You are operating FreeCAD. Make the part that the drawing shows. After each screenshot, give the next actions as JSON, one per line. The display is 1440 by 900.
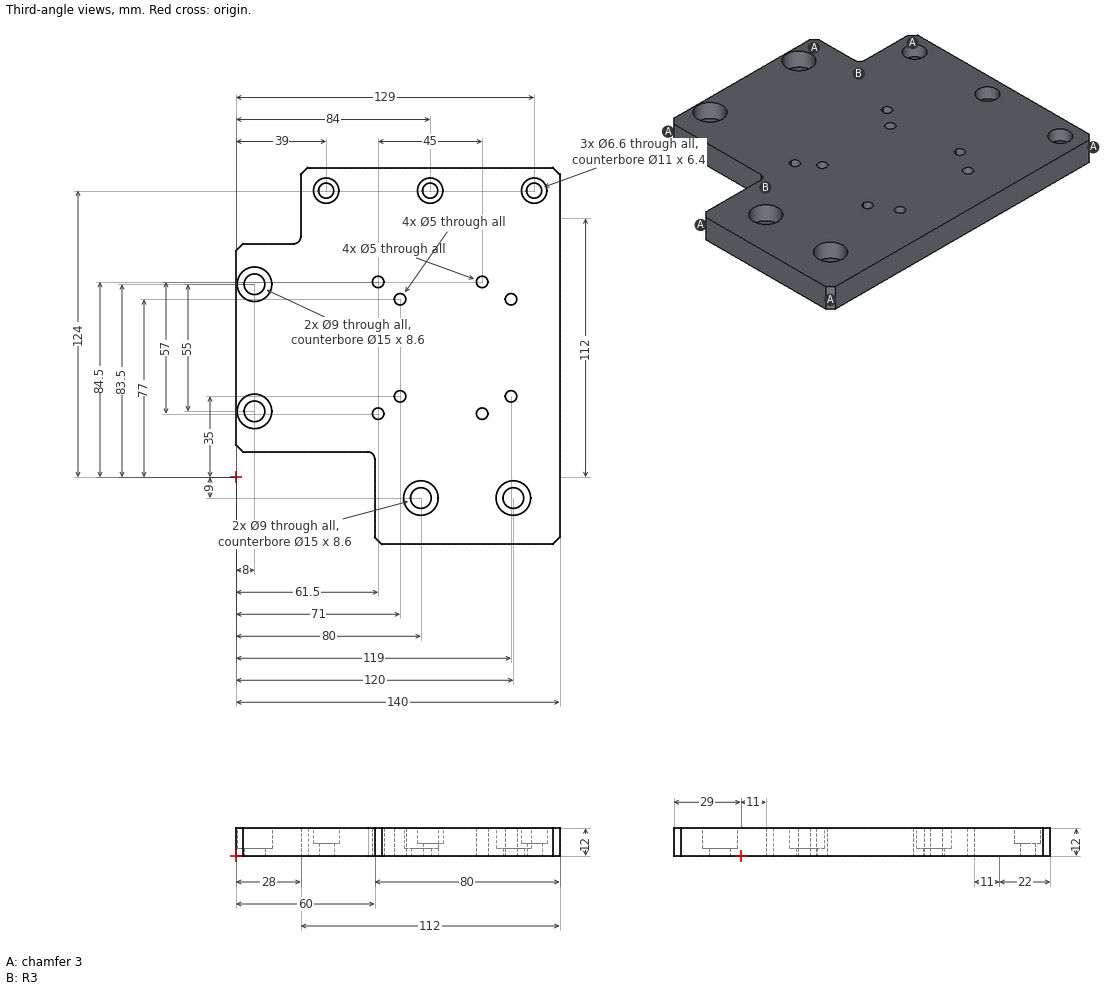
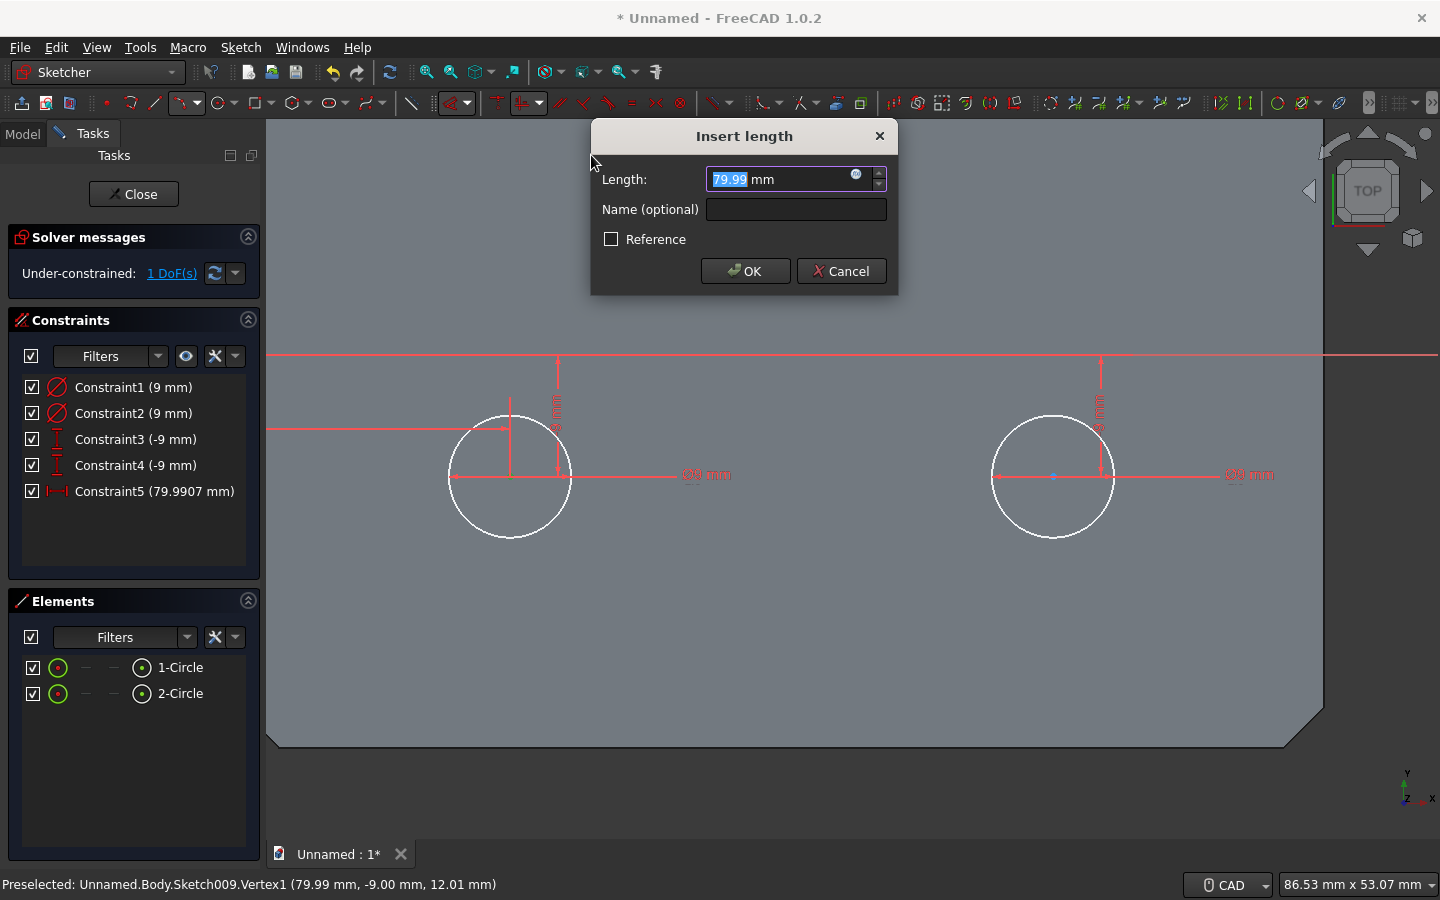
{"action": "type", "text": "80"}
{"action": "key", "text": "Return"}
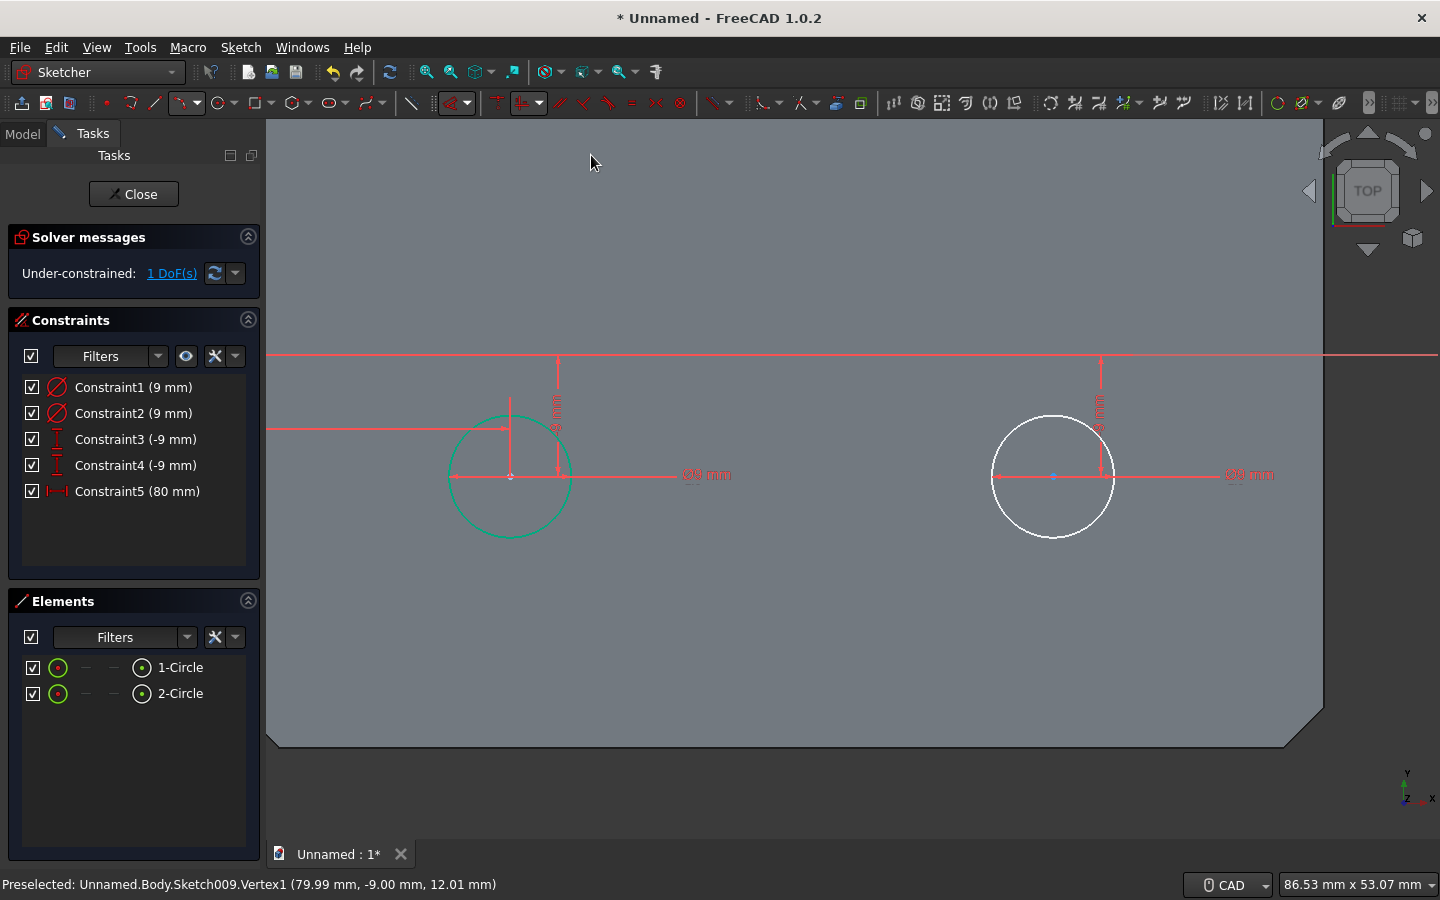
{"action": "left_click", "coordinate": [1053, 477]}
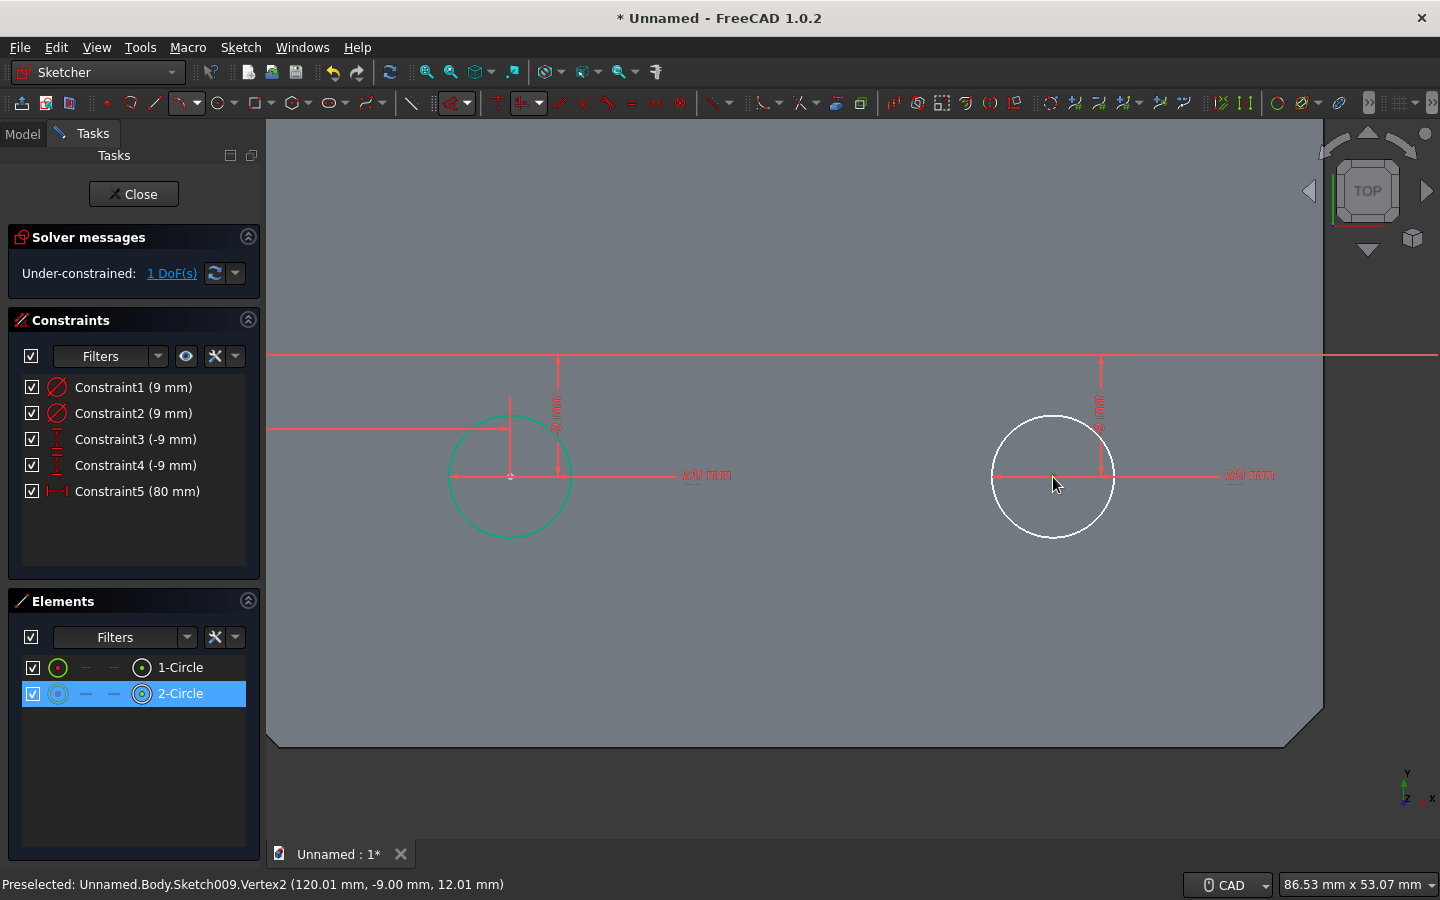
{"action": "key", "text": "l"}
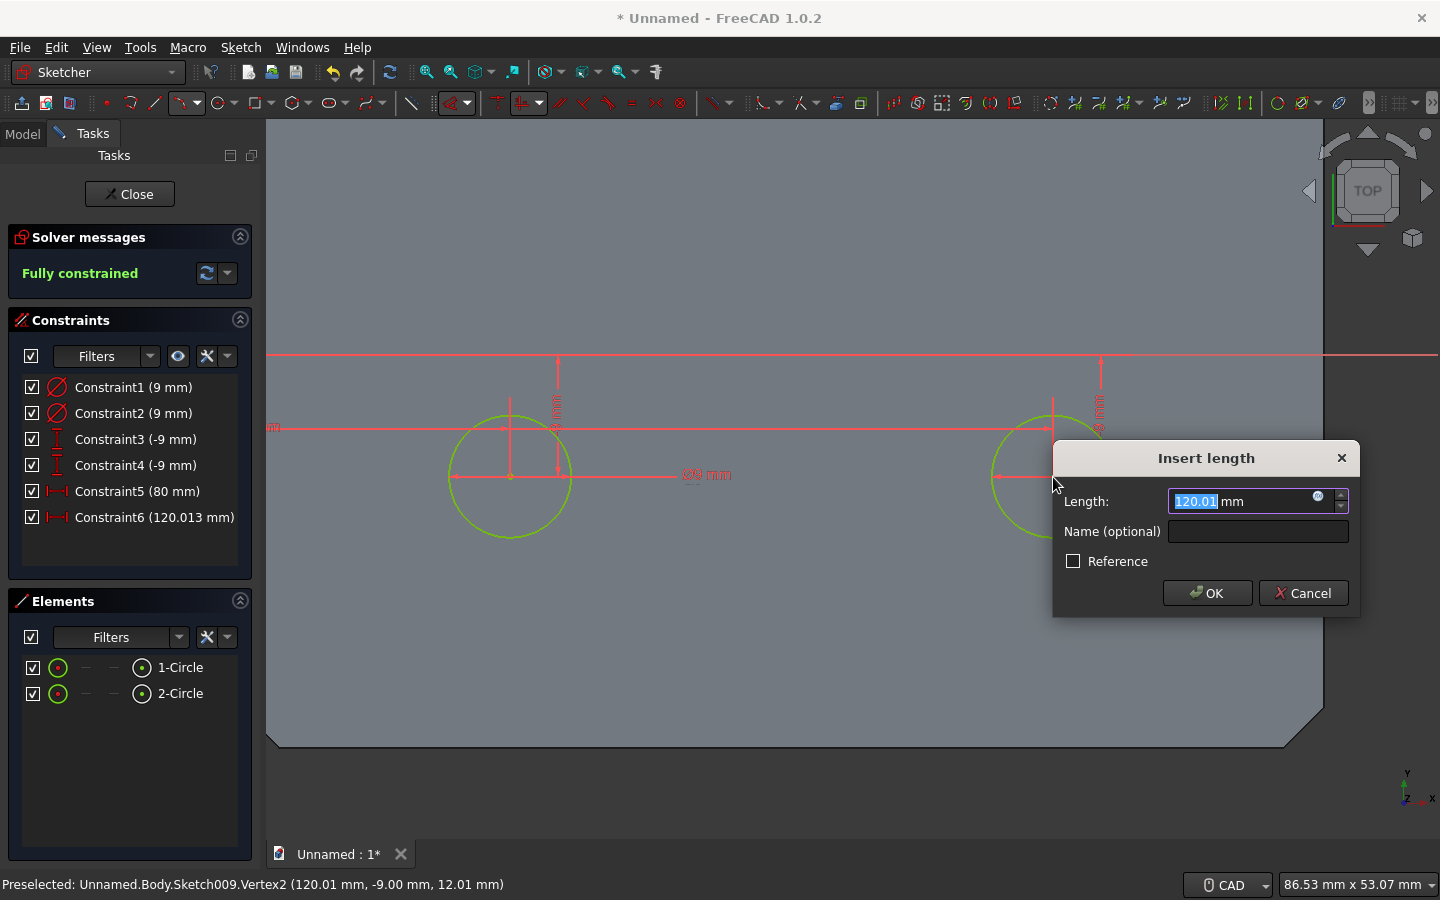
{"action": "type", "text": "120"}
{"action": "key", "text": "Return"}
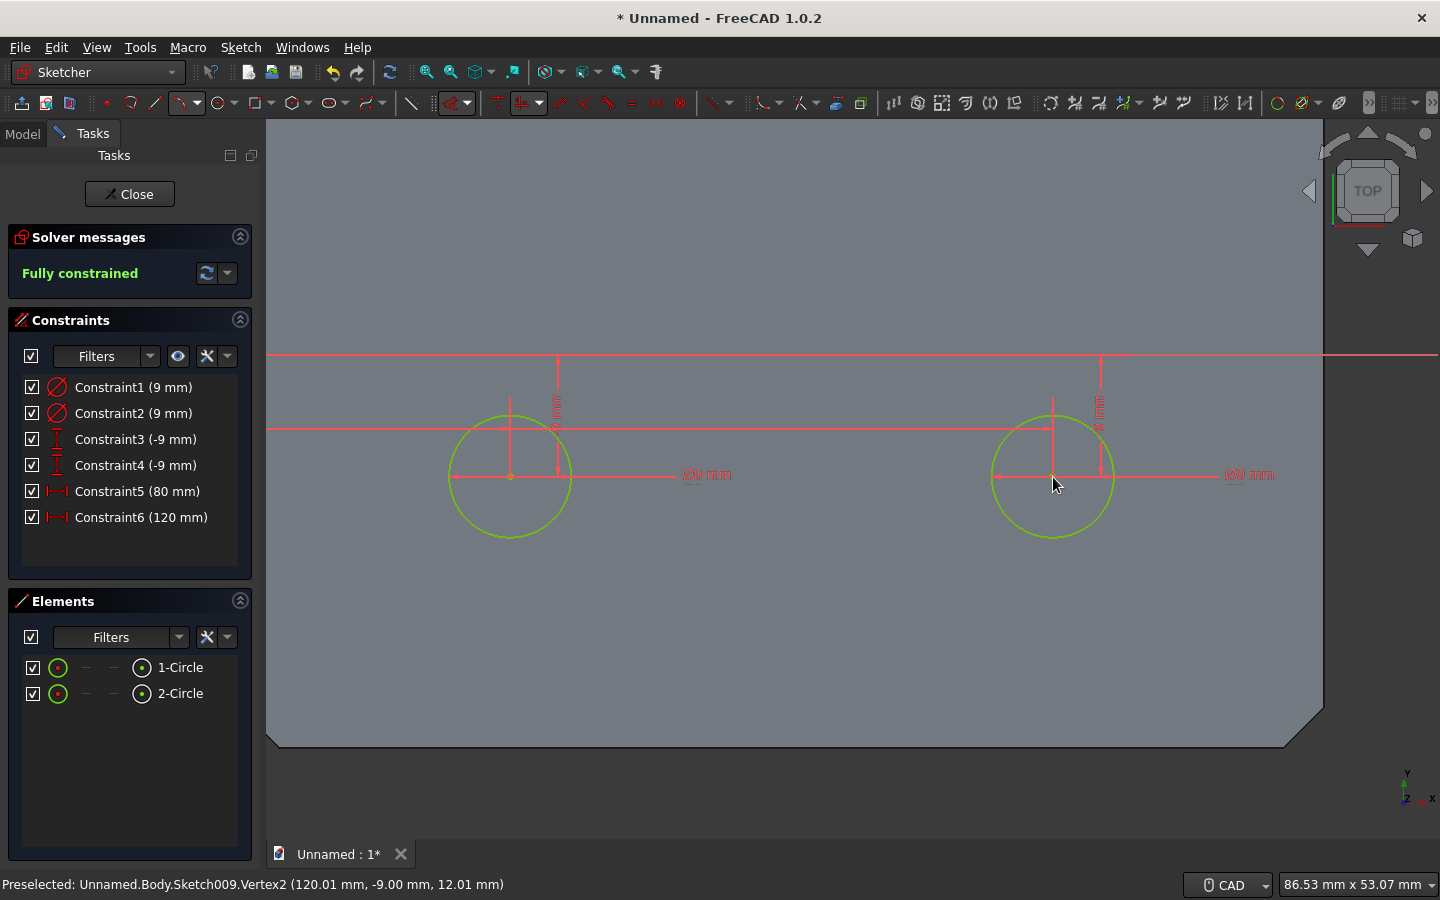
{"action": "left_click", "coordinate": [130, 194]}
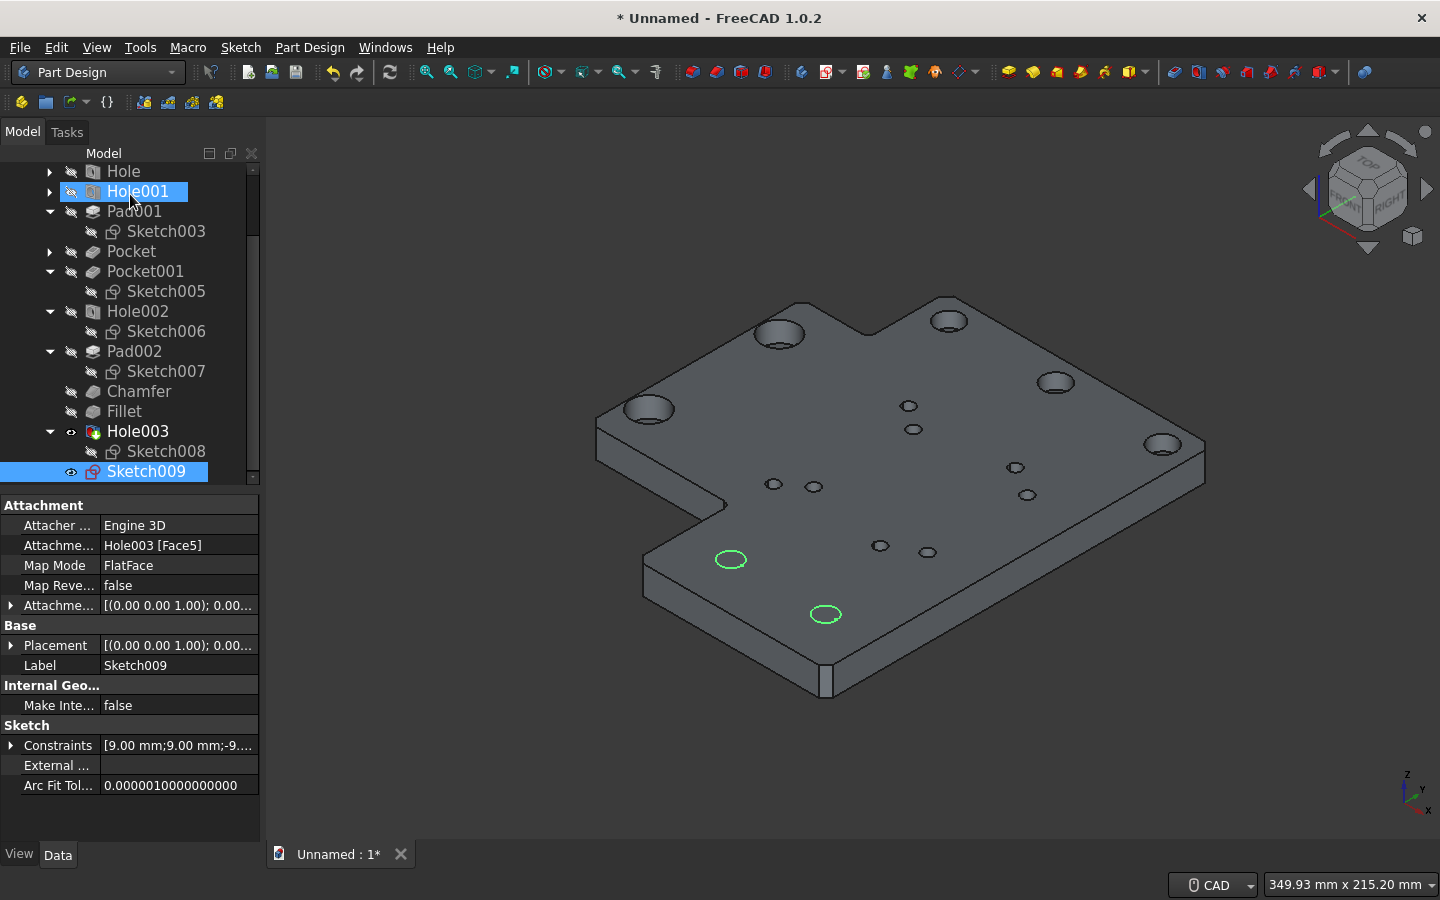
{"action": "left_click", "coordinate": [1200, 72]}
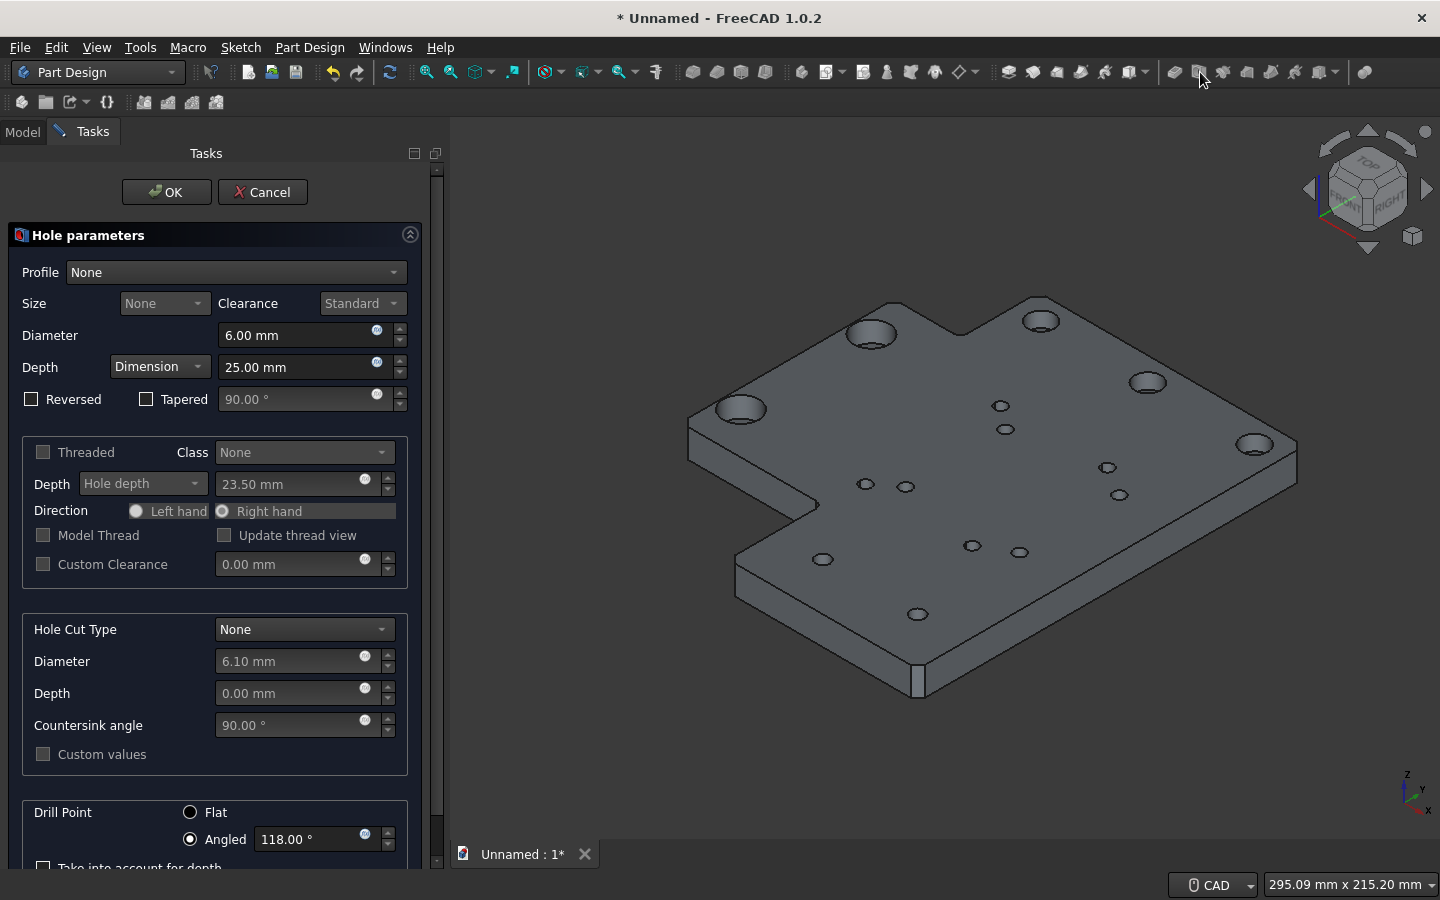
{"action": "triple_click", "coordinate": [305, 335]}